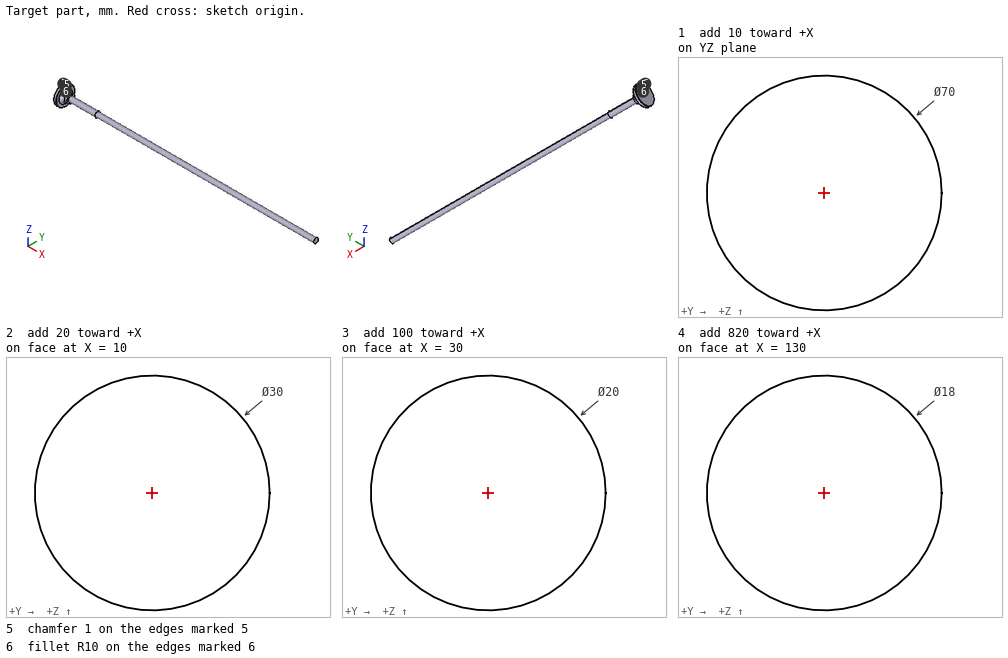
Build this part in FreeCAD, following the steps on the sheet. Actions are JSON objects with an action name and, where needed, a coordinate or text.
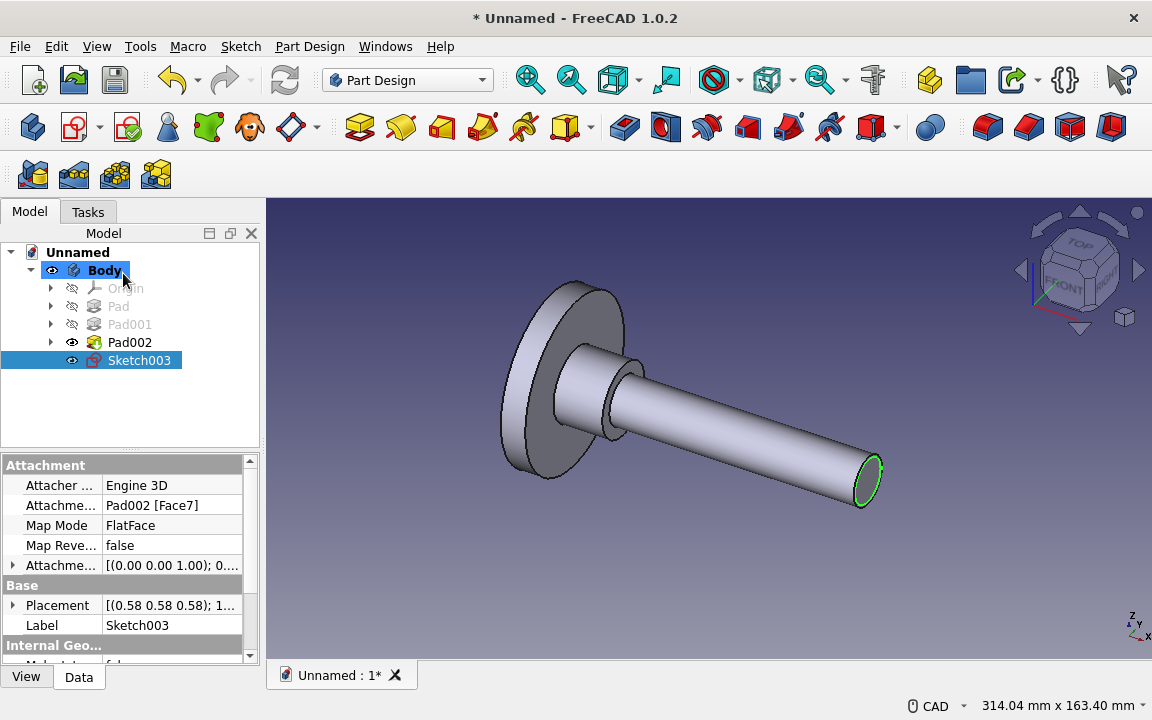
{"action": "left_click", "coordinate": [360, 128]}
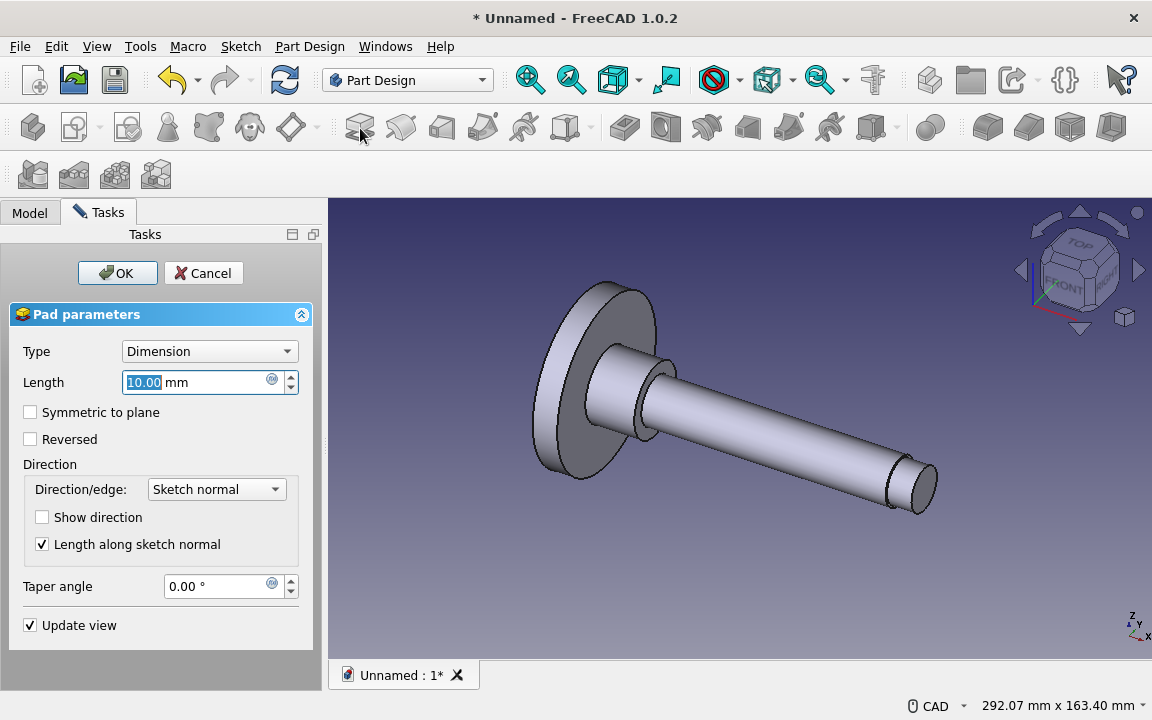
{"action": "type", "text": "820"}
{"action": "key", "text": "Tab"}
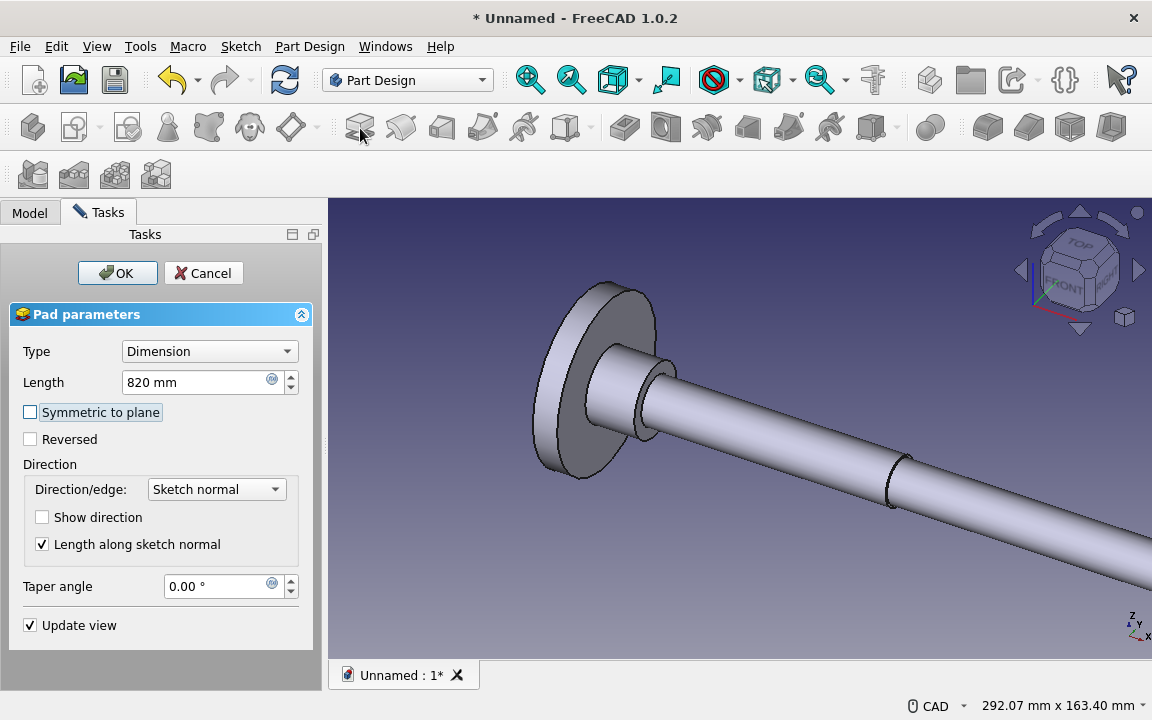
{"action": "left_click", "coordinate": [118, 273]}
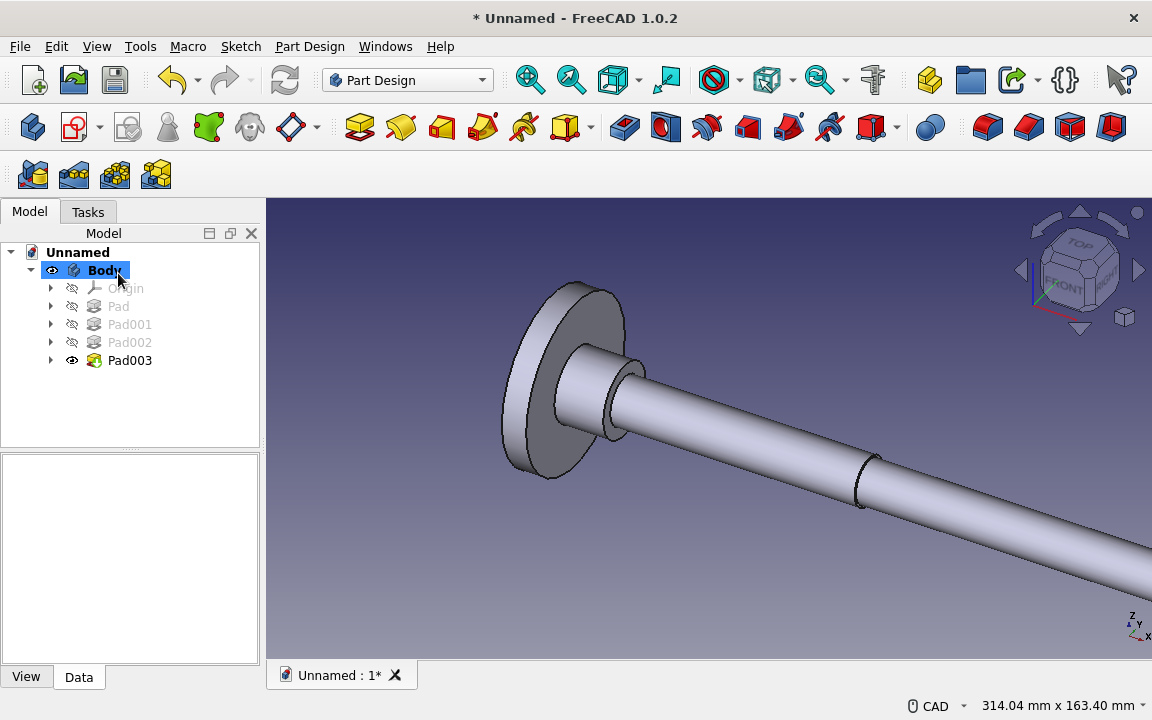
{"action": "key", "text": "v f"}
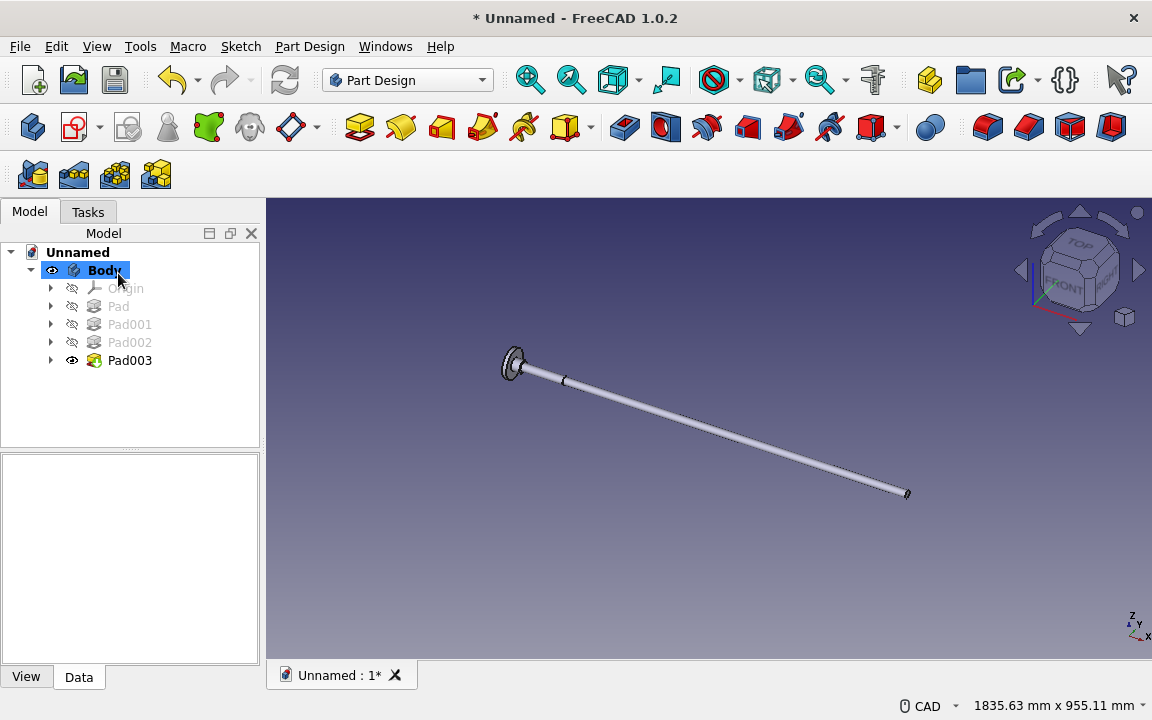
{"action": "left_click", "coordinate": [506, 372]}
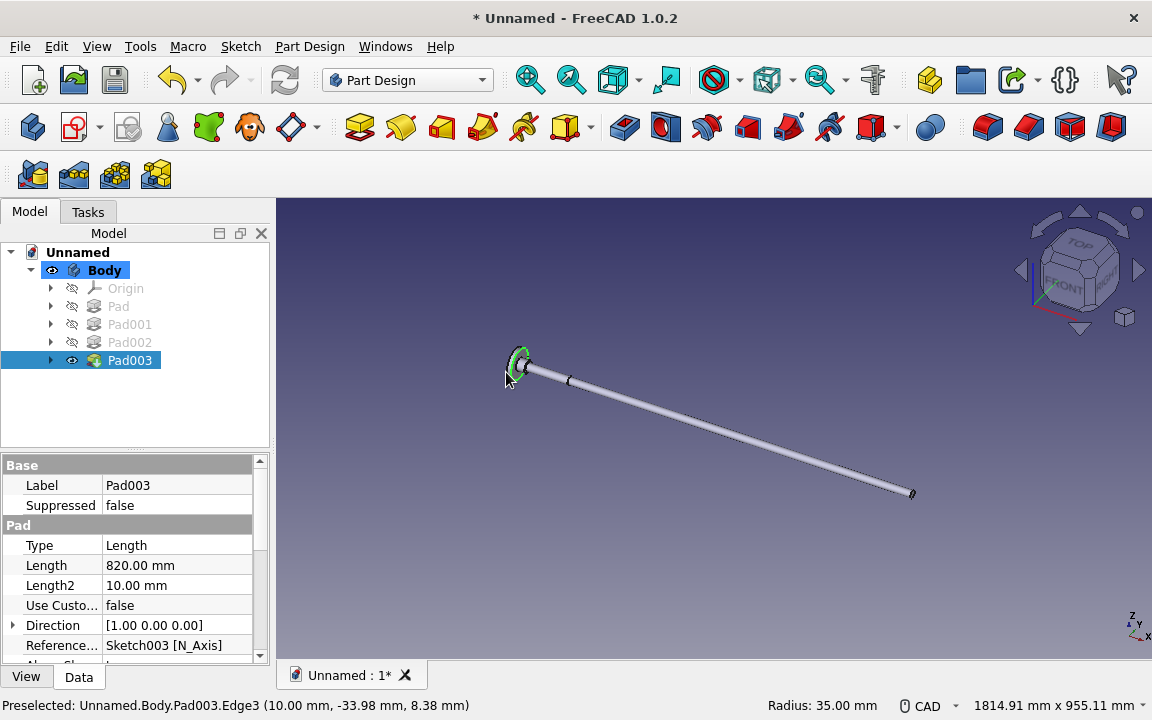
{"action": "key", "text": "0"}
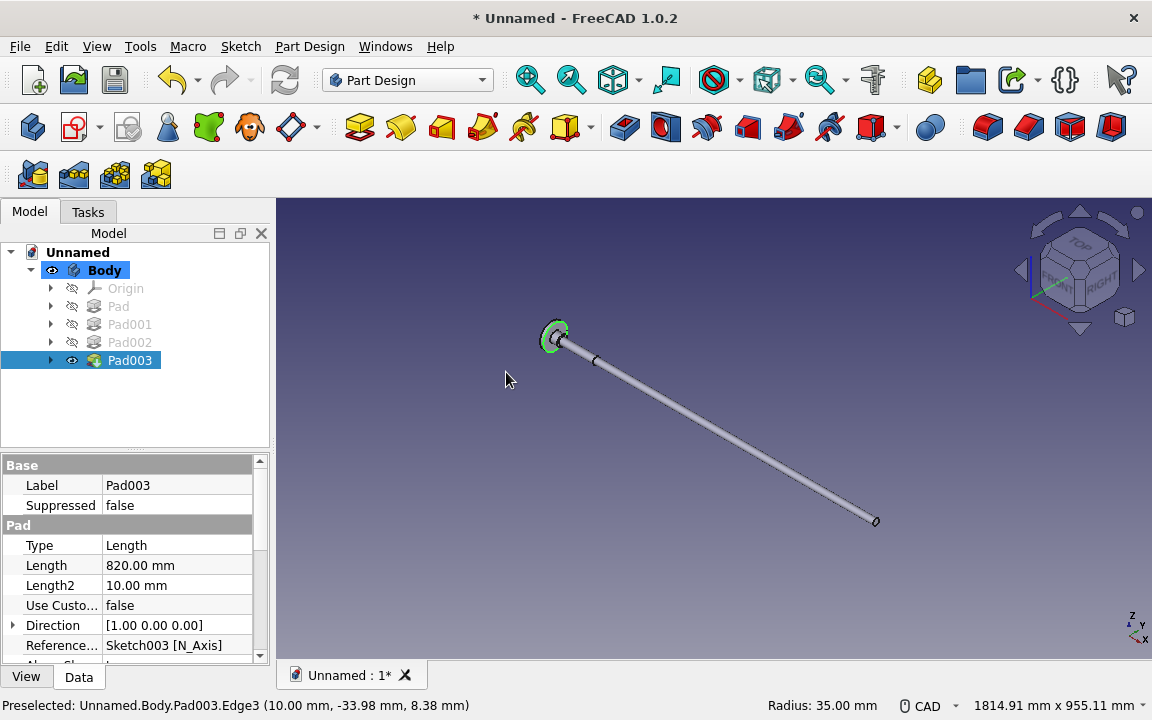
{"action": "key", "text": "2"}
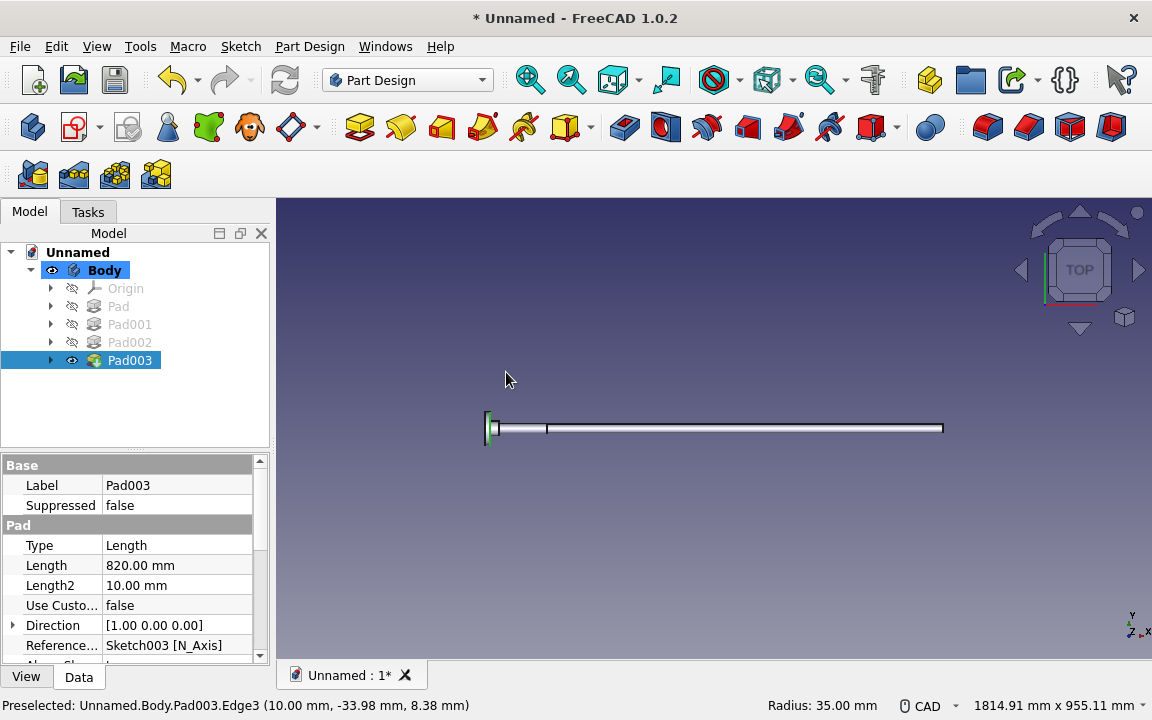
{"action": "left_click", "coordinate": [485, 444], "text": "ctrl"}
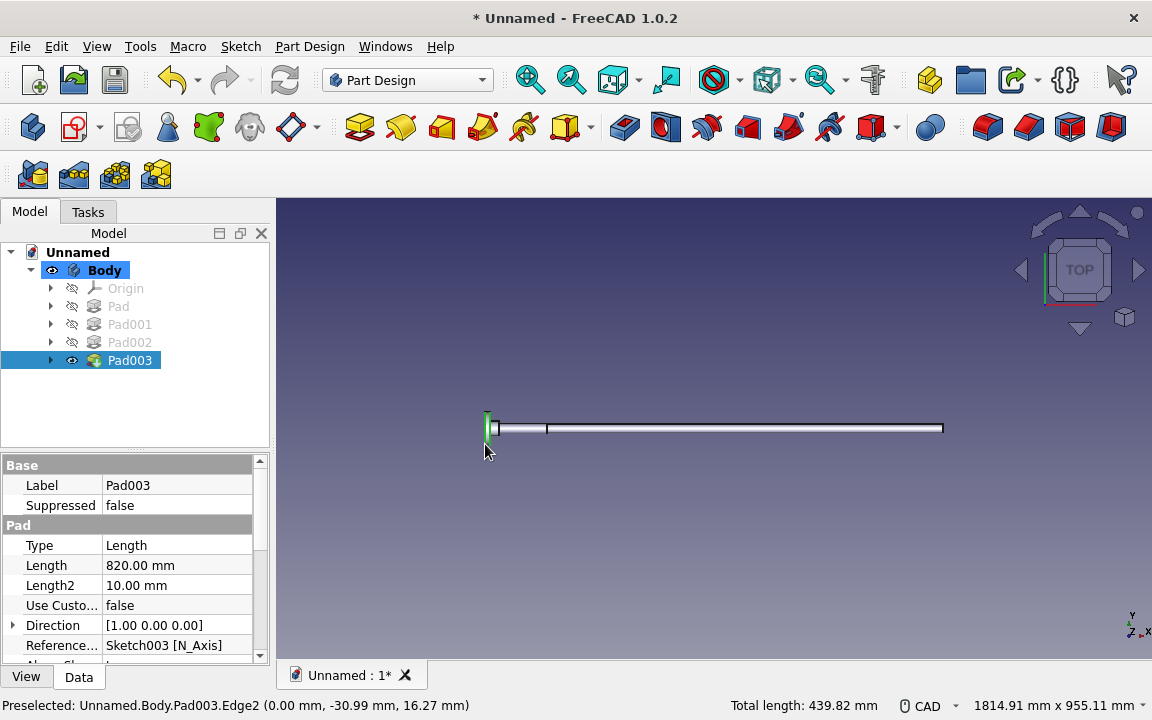
{"action": "left_click", "coordinate": [1029, 128]}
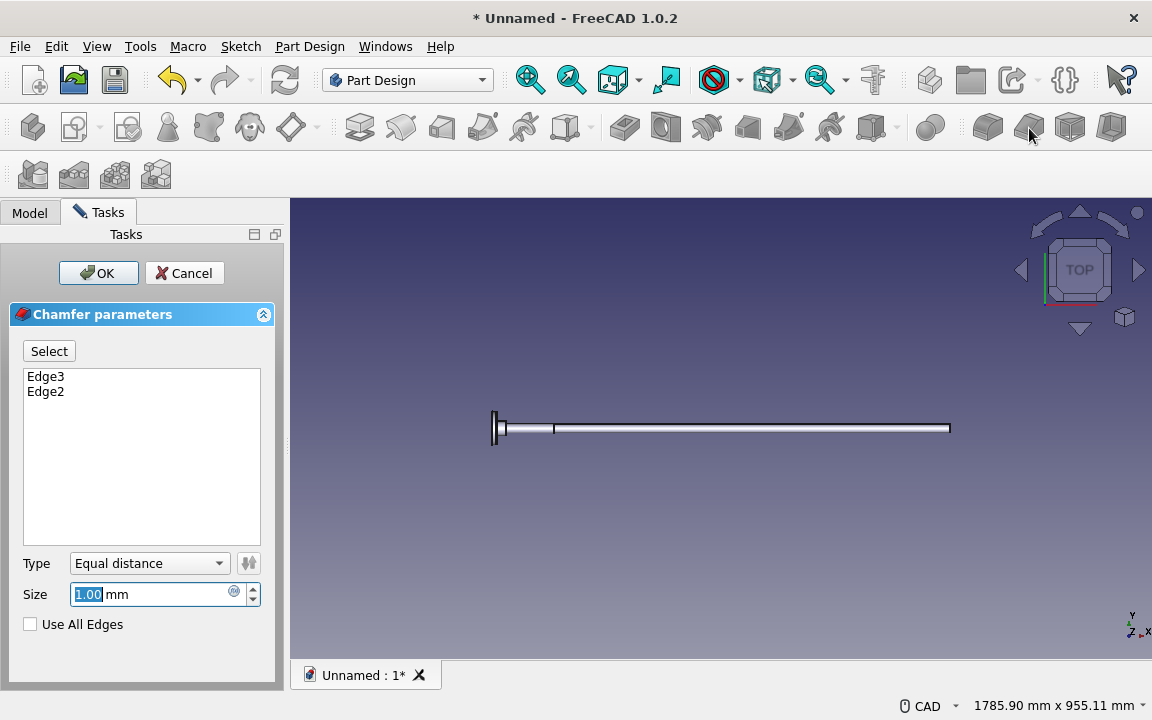
{"action": "type", "text": "1"}
{"action": "key", "text": "Tab"}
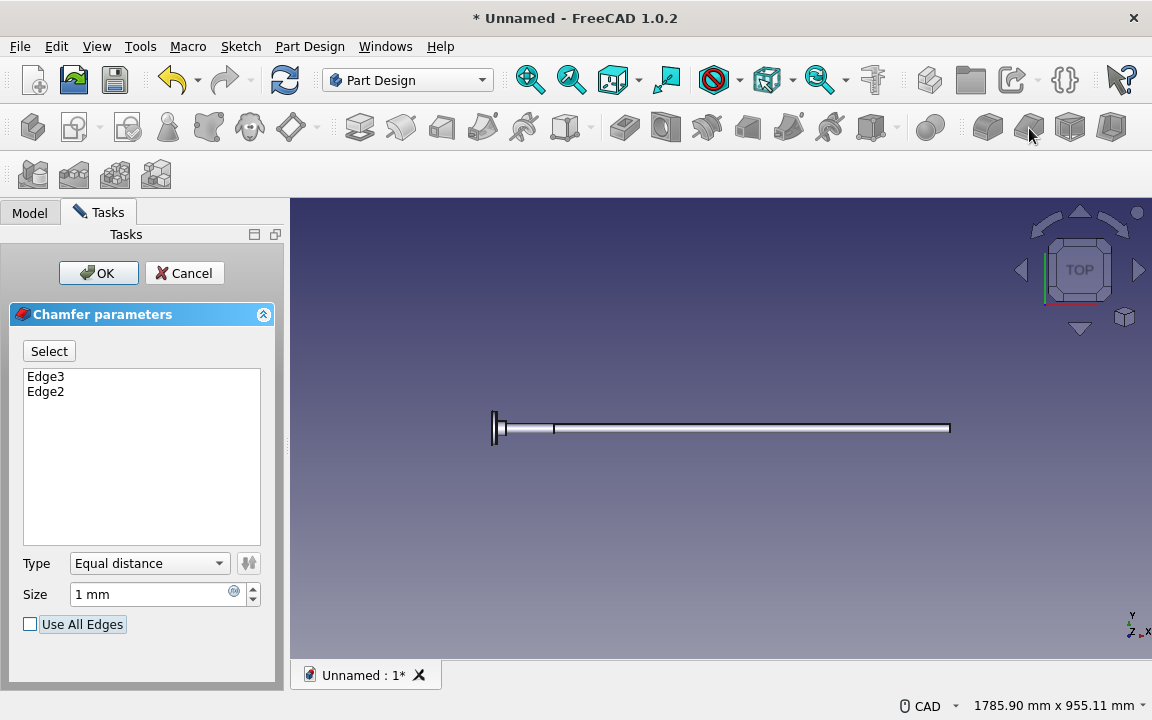
{"action": "left_click", "coordinate": [99, 273]}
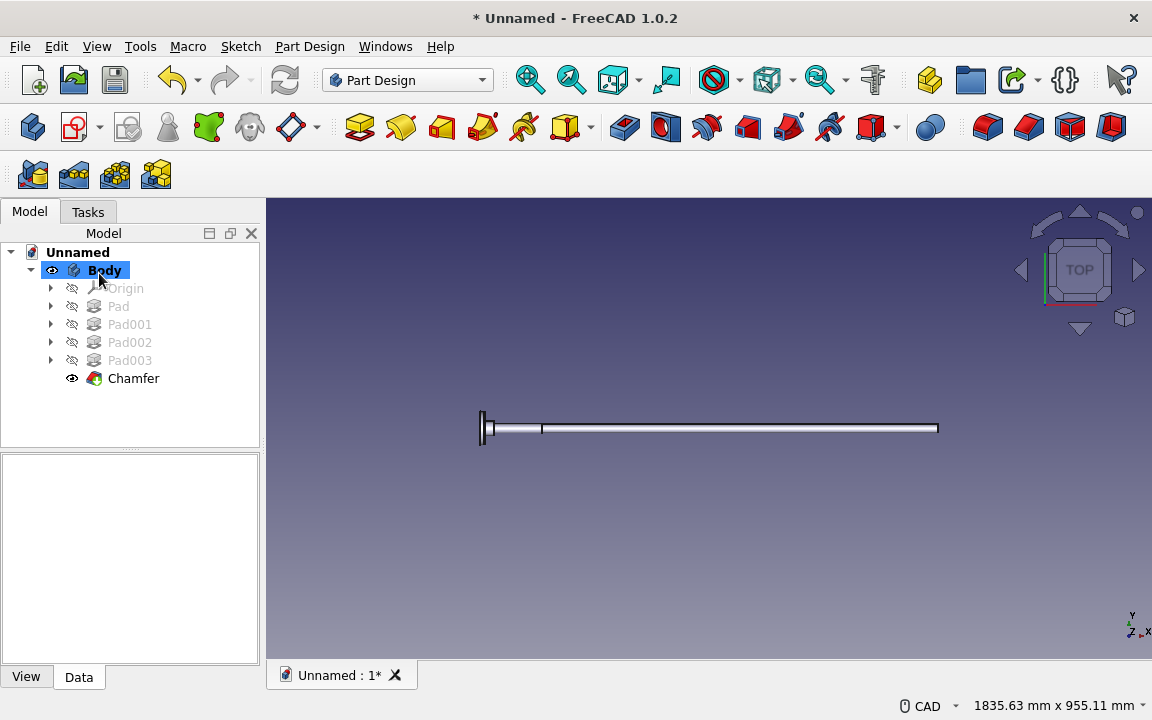
{"action": "key", "text": "0"}